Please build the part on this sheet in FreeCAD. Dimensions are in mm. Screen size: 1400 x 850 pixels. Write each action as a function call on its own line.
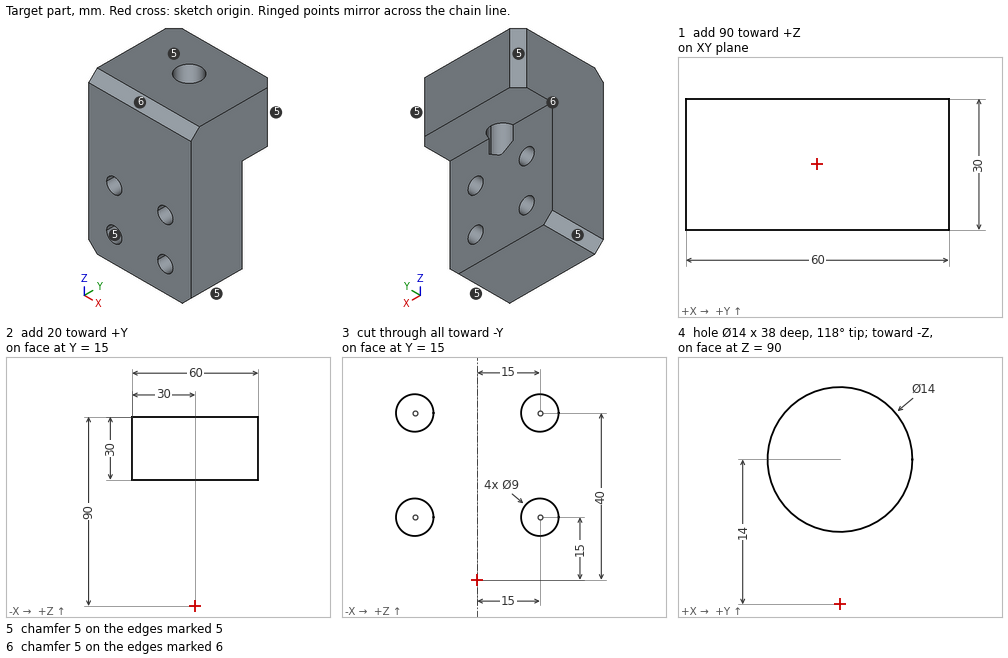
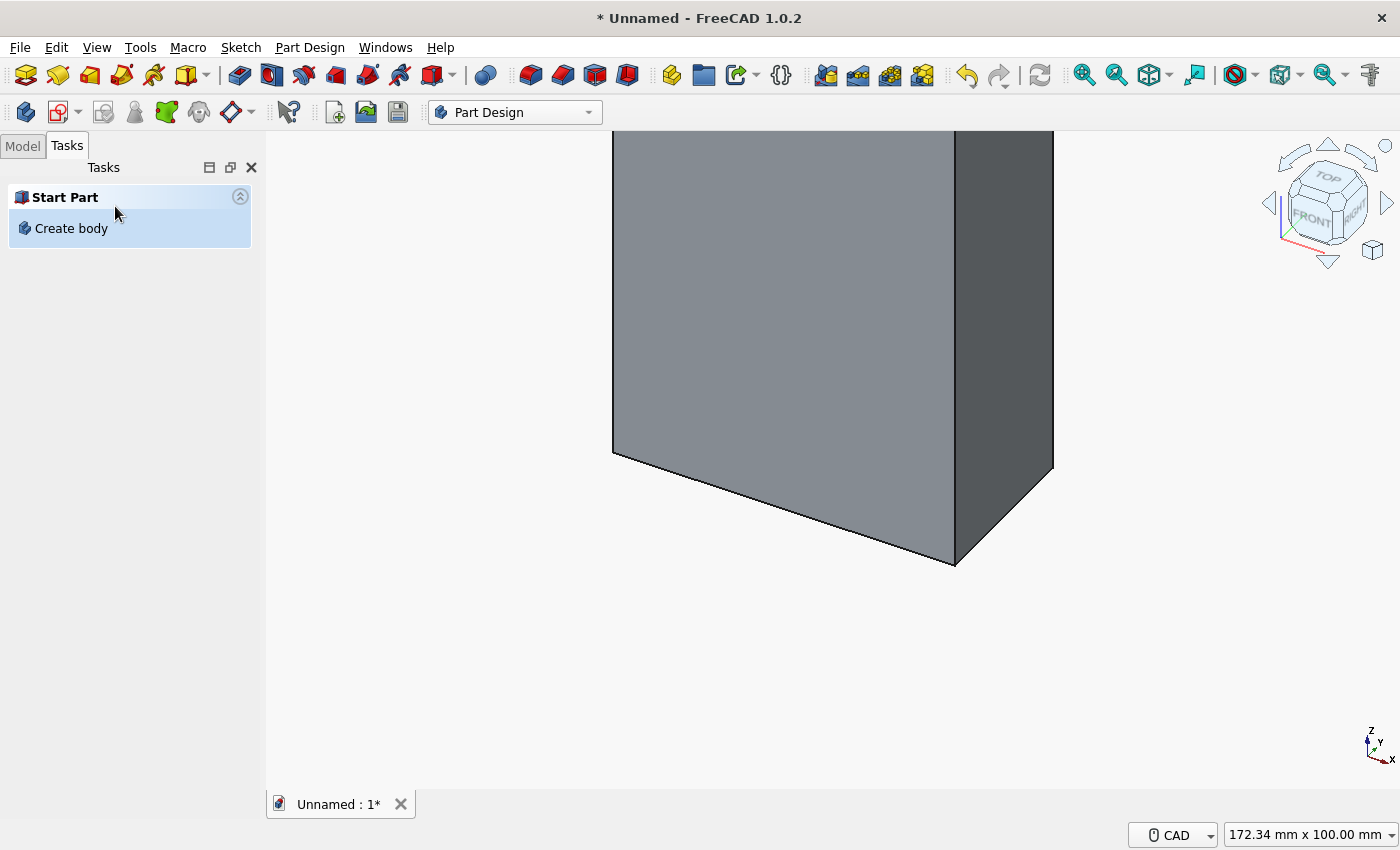
click(1086, 76)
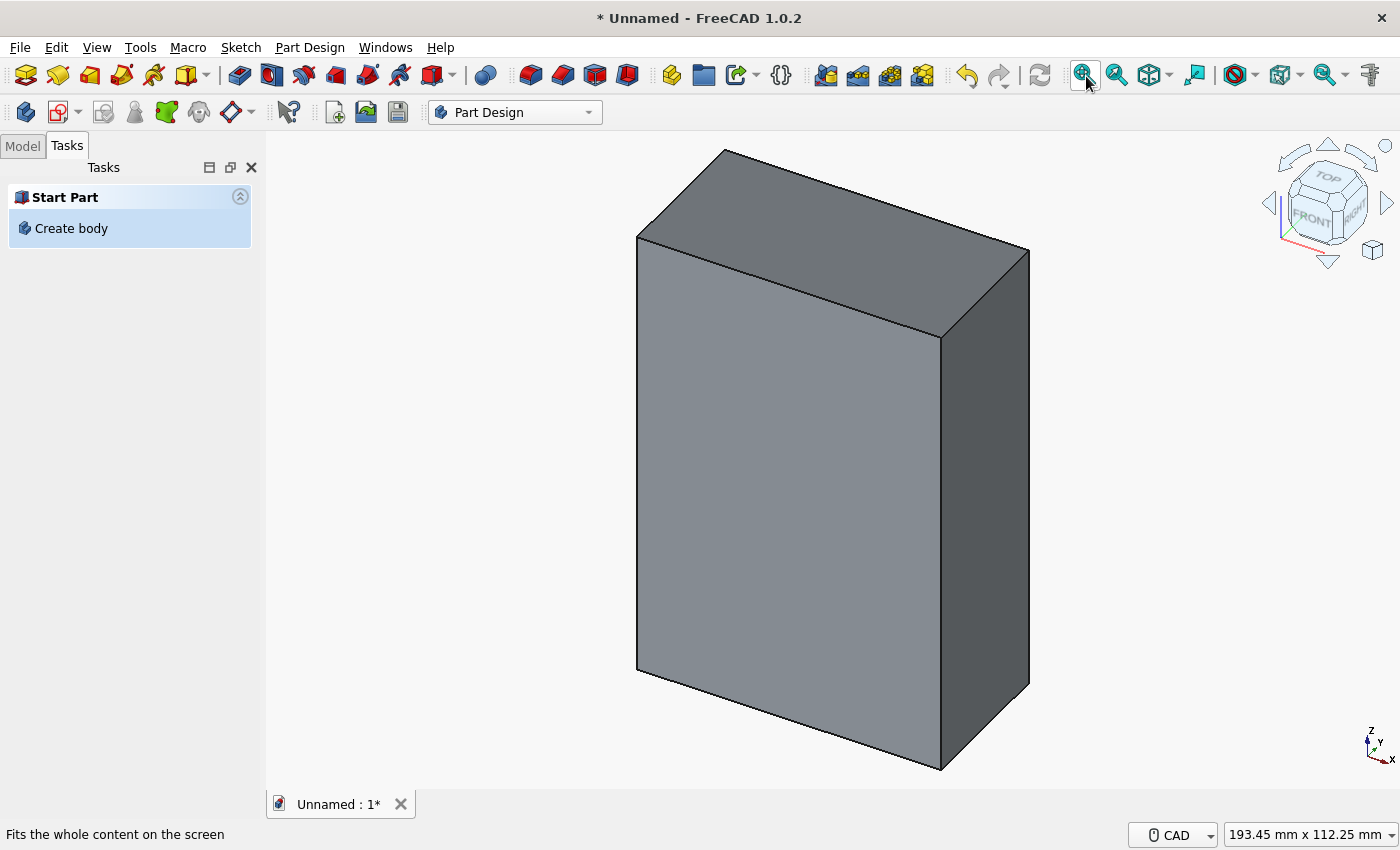
key(4)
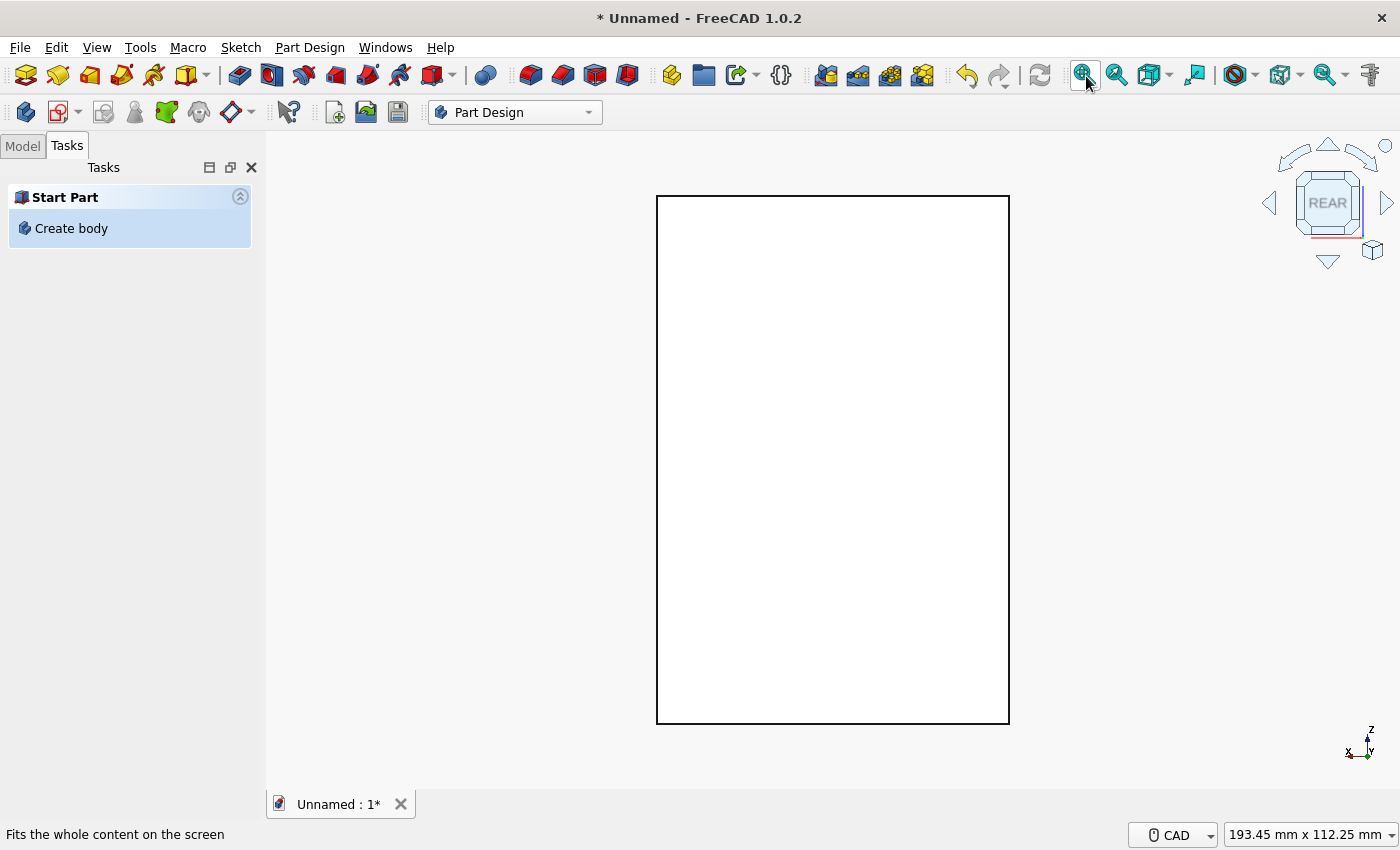
click(833, 384)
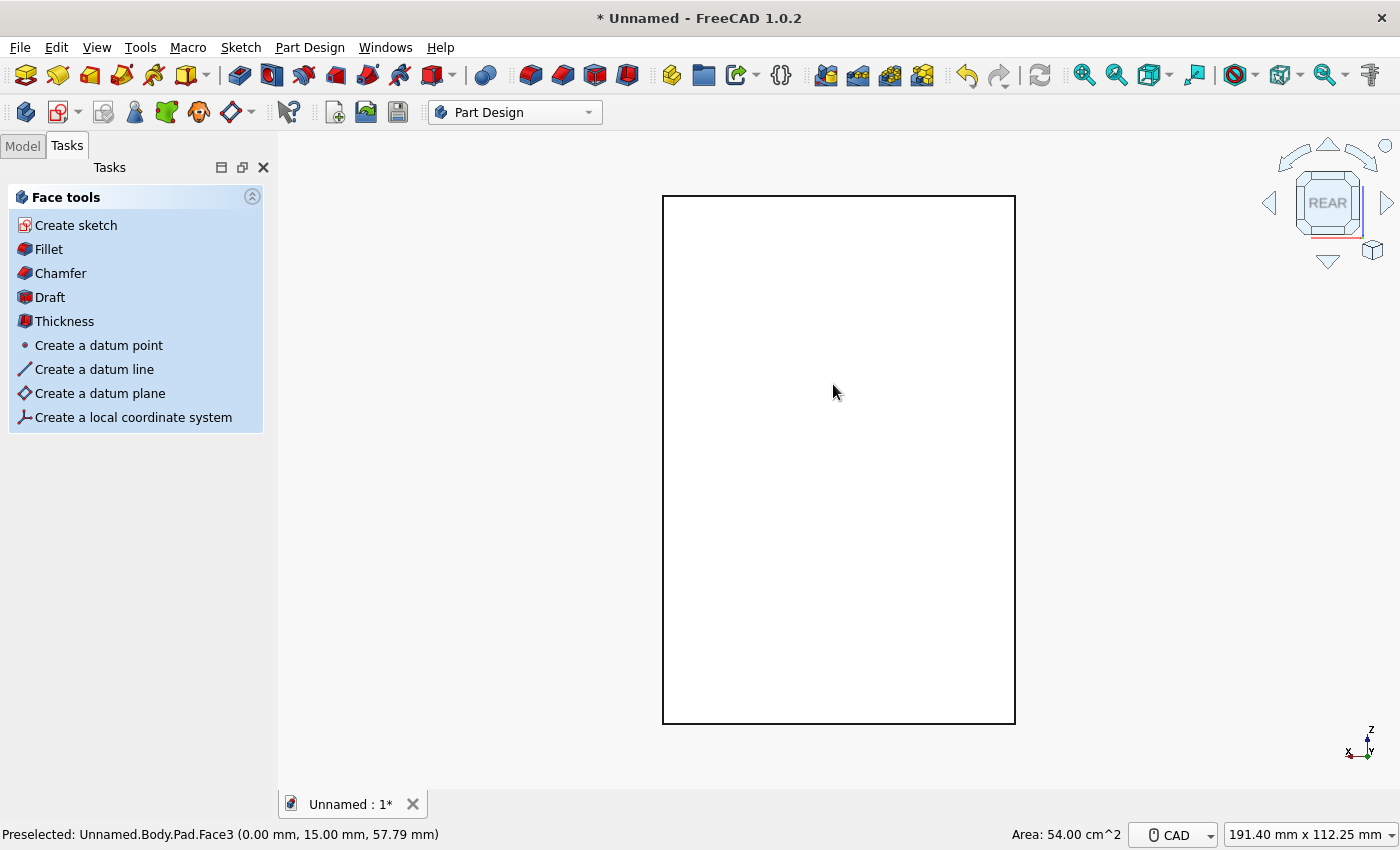
click(58, 112)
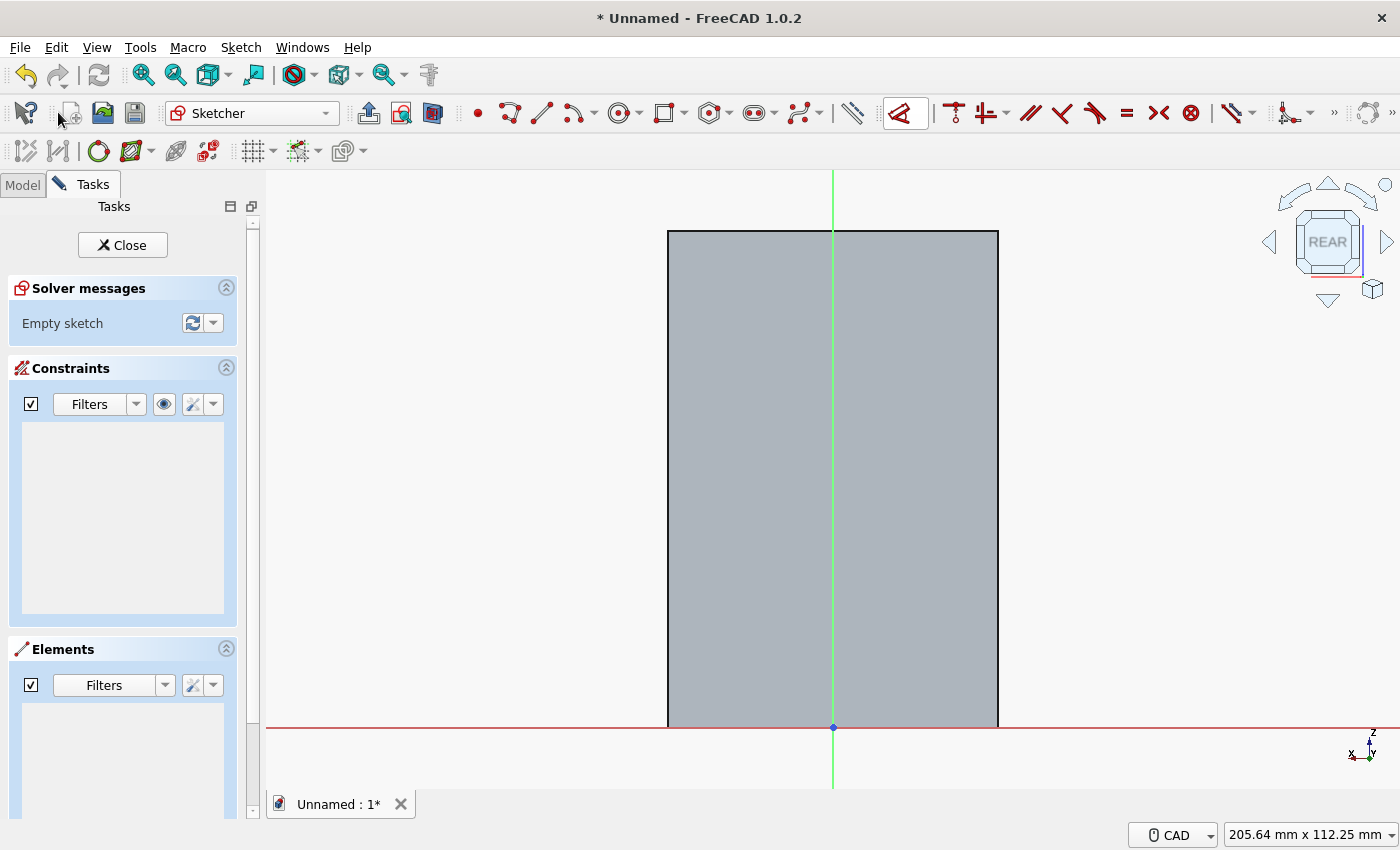
click(664, 114)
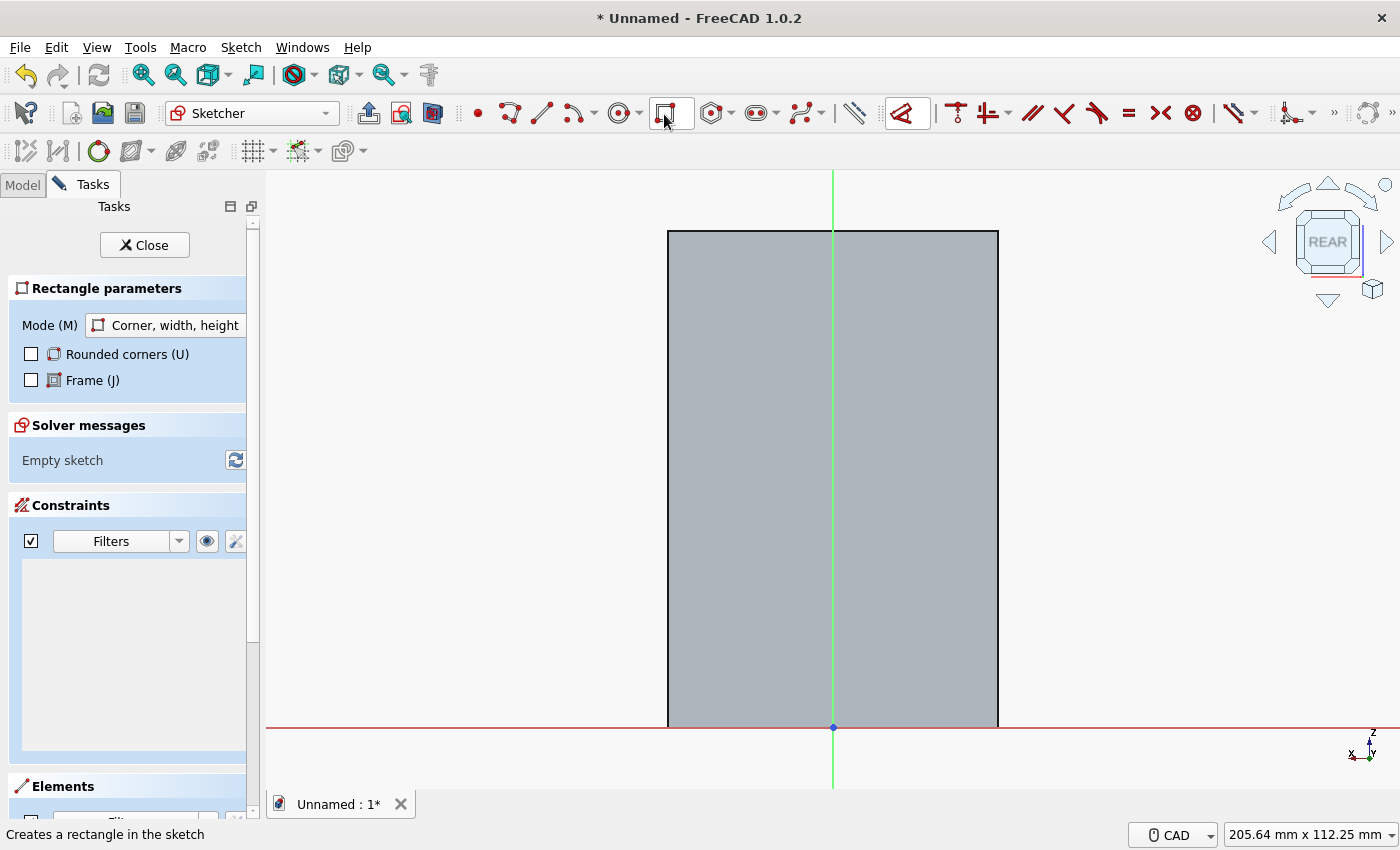
click(668, 231)
click(998, 397)
key(Escape)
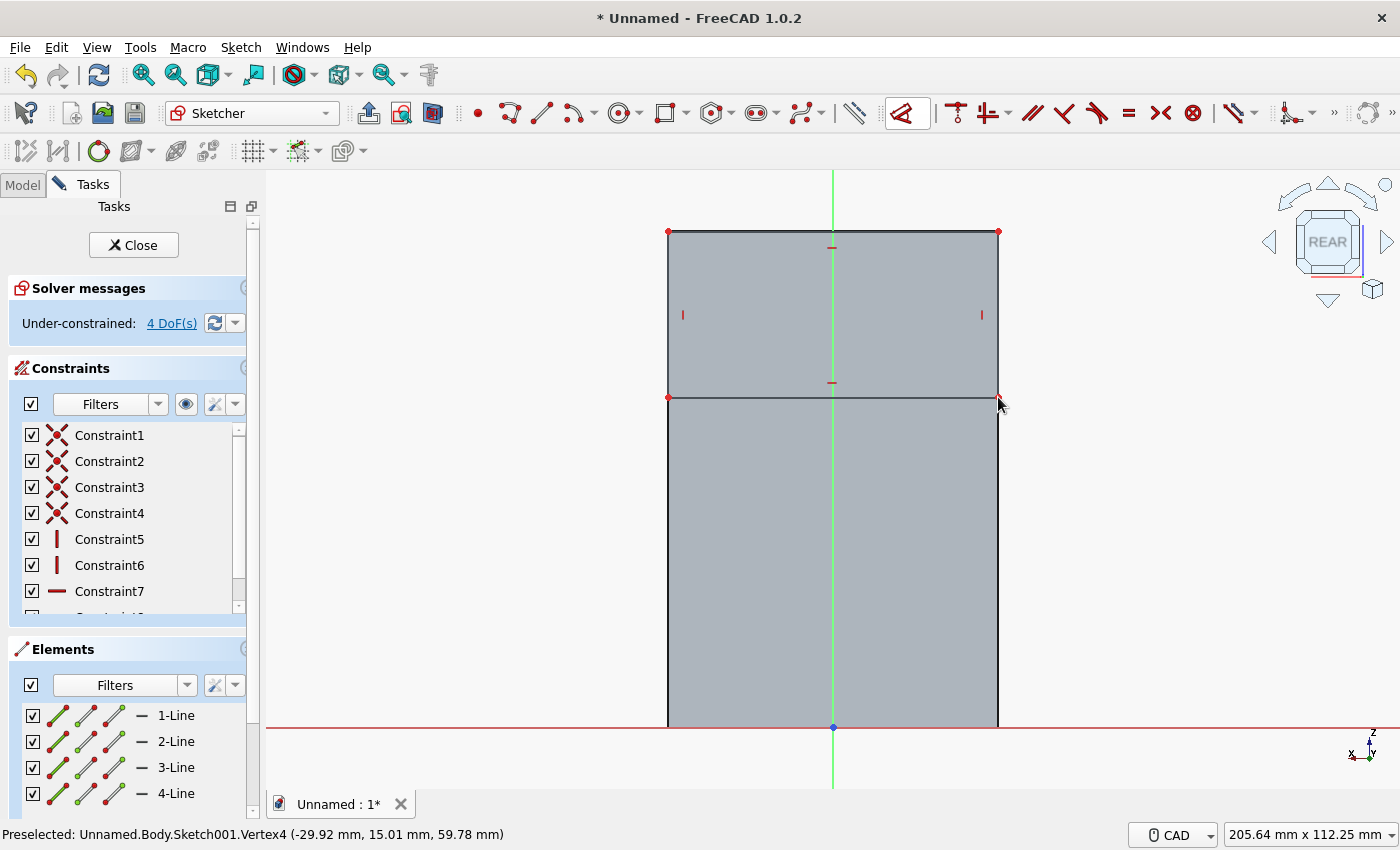
click(668, 282)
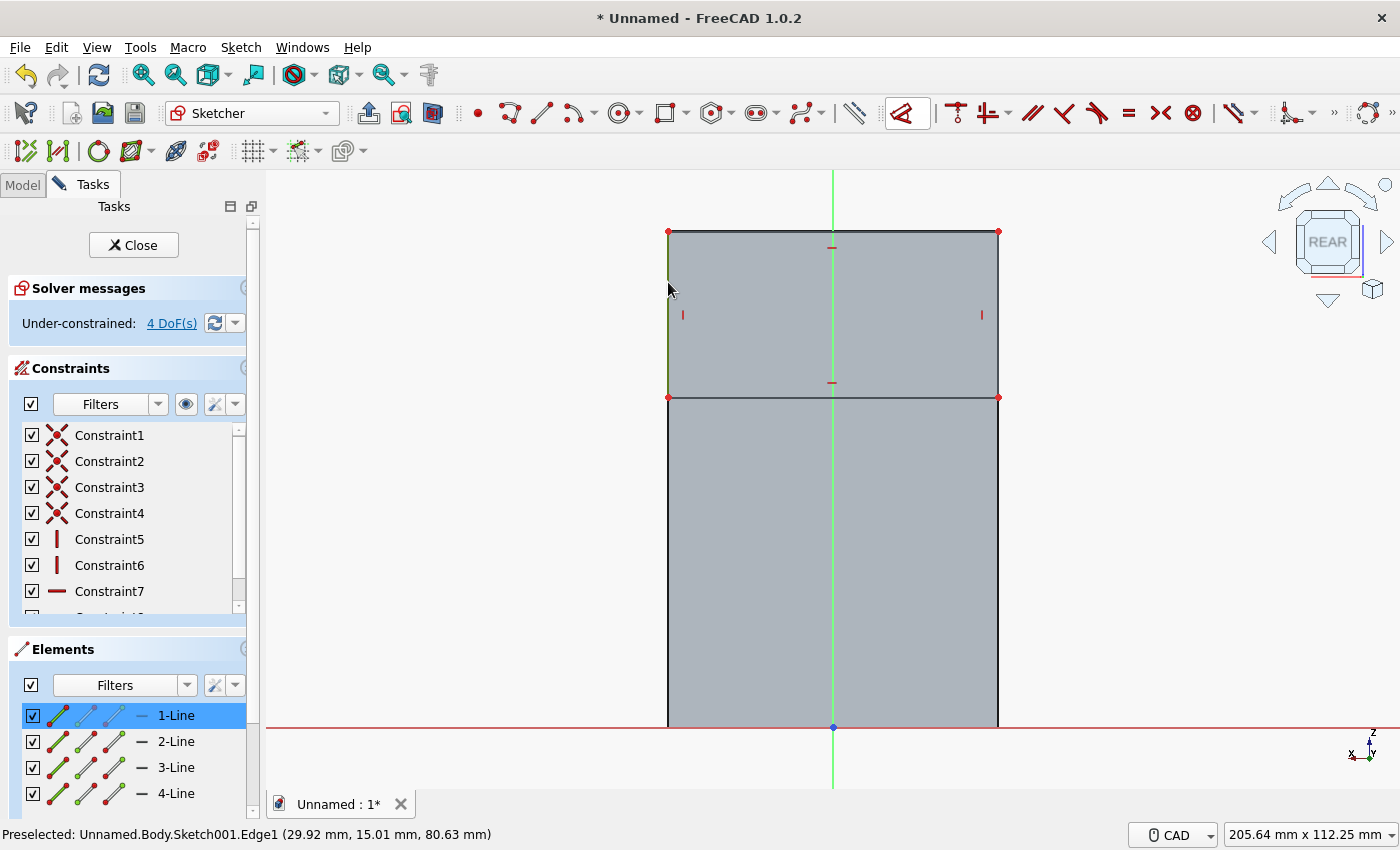
key(i)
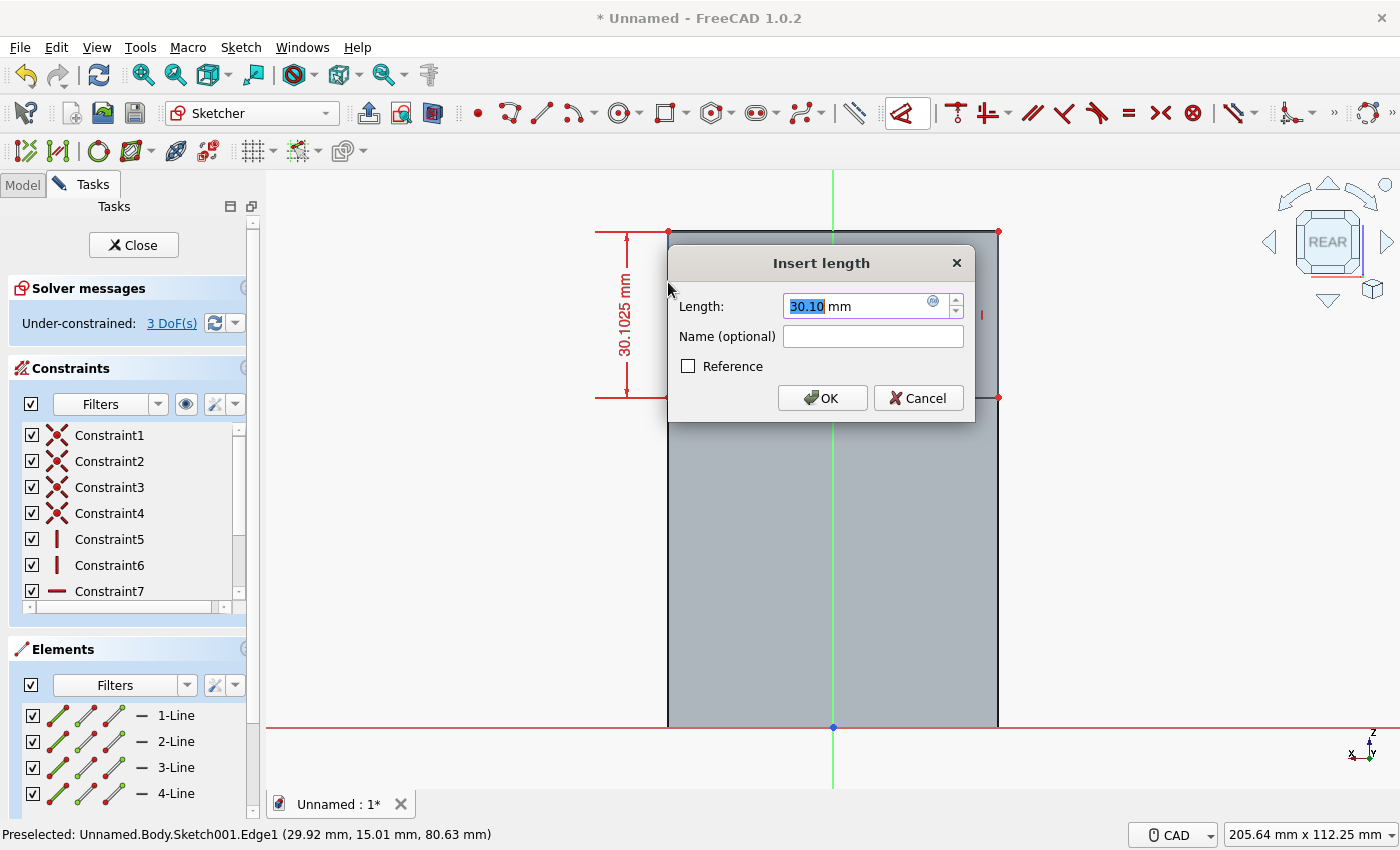
text(30)
key(Return)